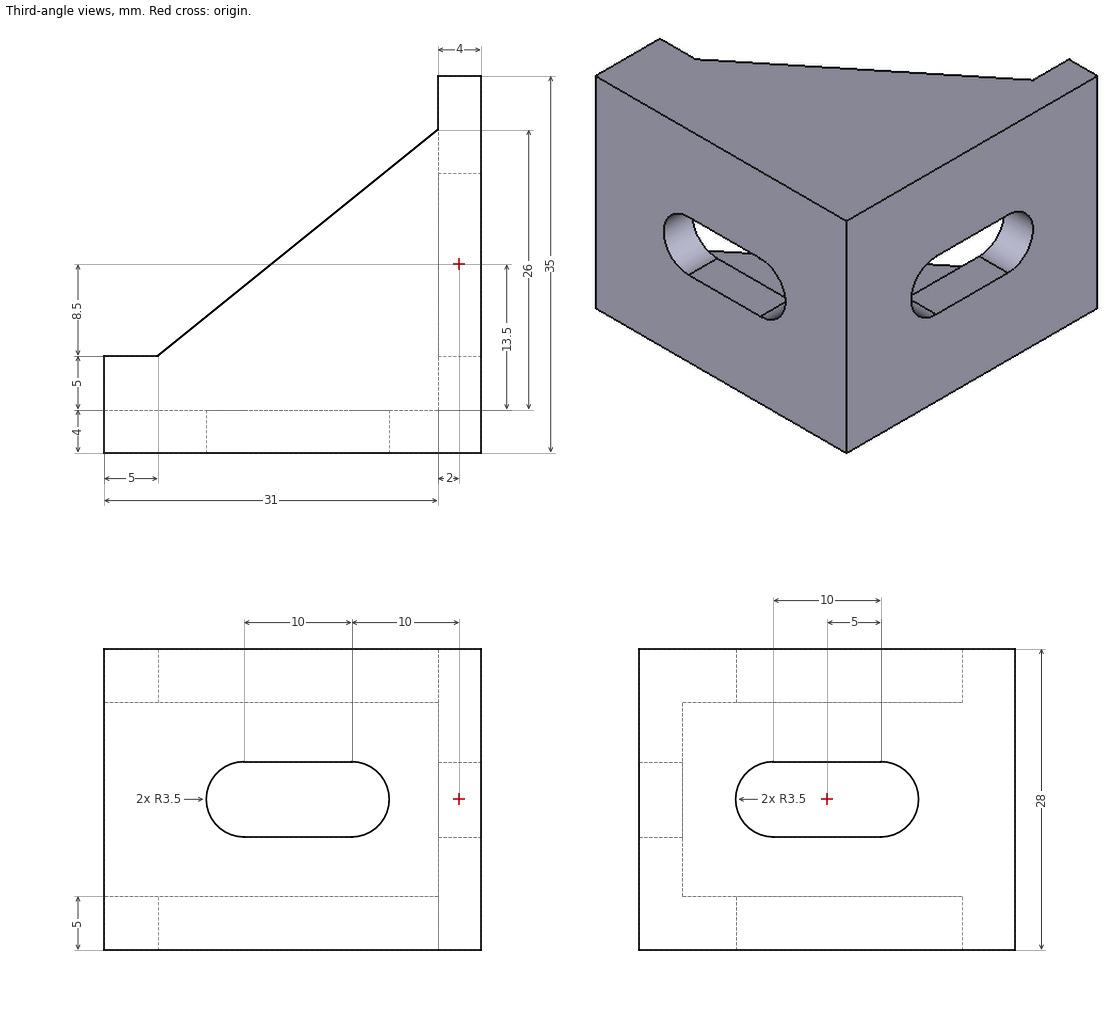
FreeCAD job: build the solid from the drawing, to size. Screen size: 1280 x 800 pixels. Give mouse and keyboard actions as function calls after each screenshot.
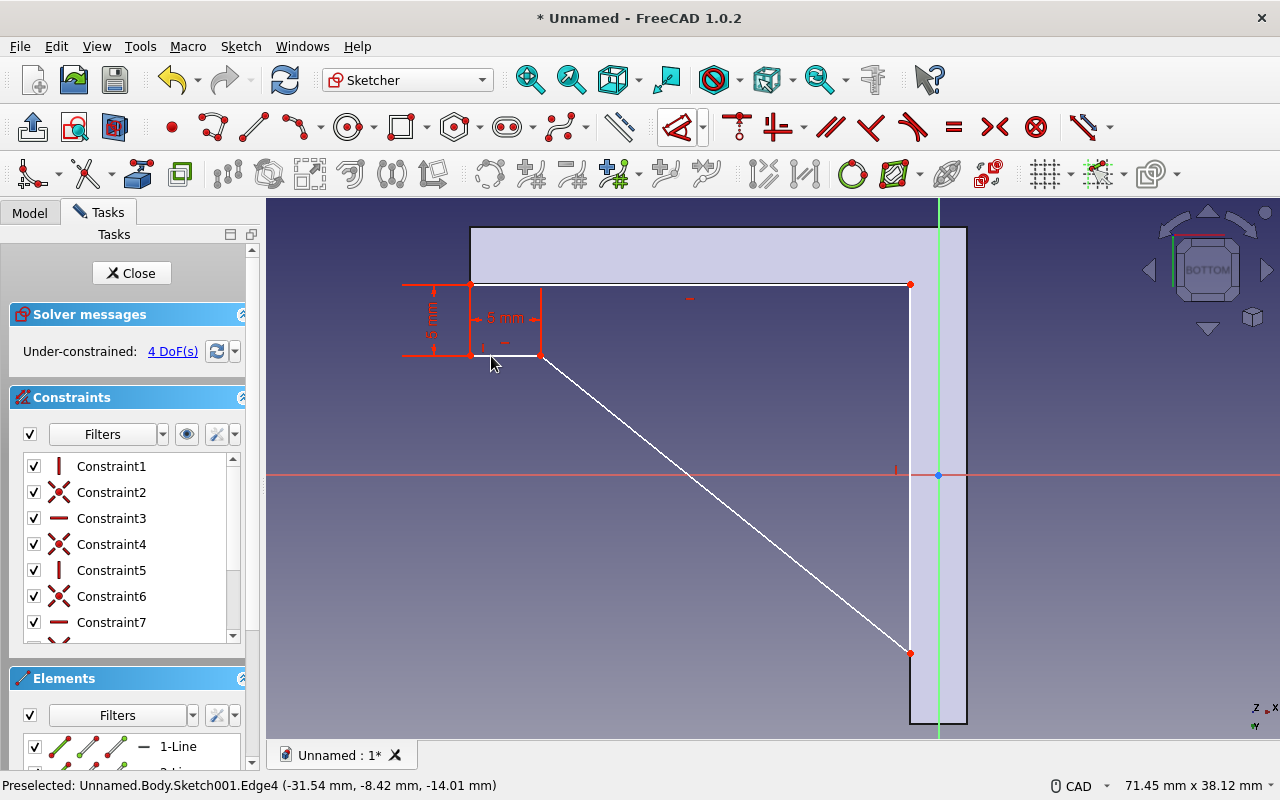
click(910, 543)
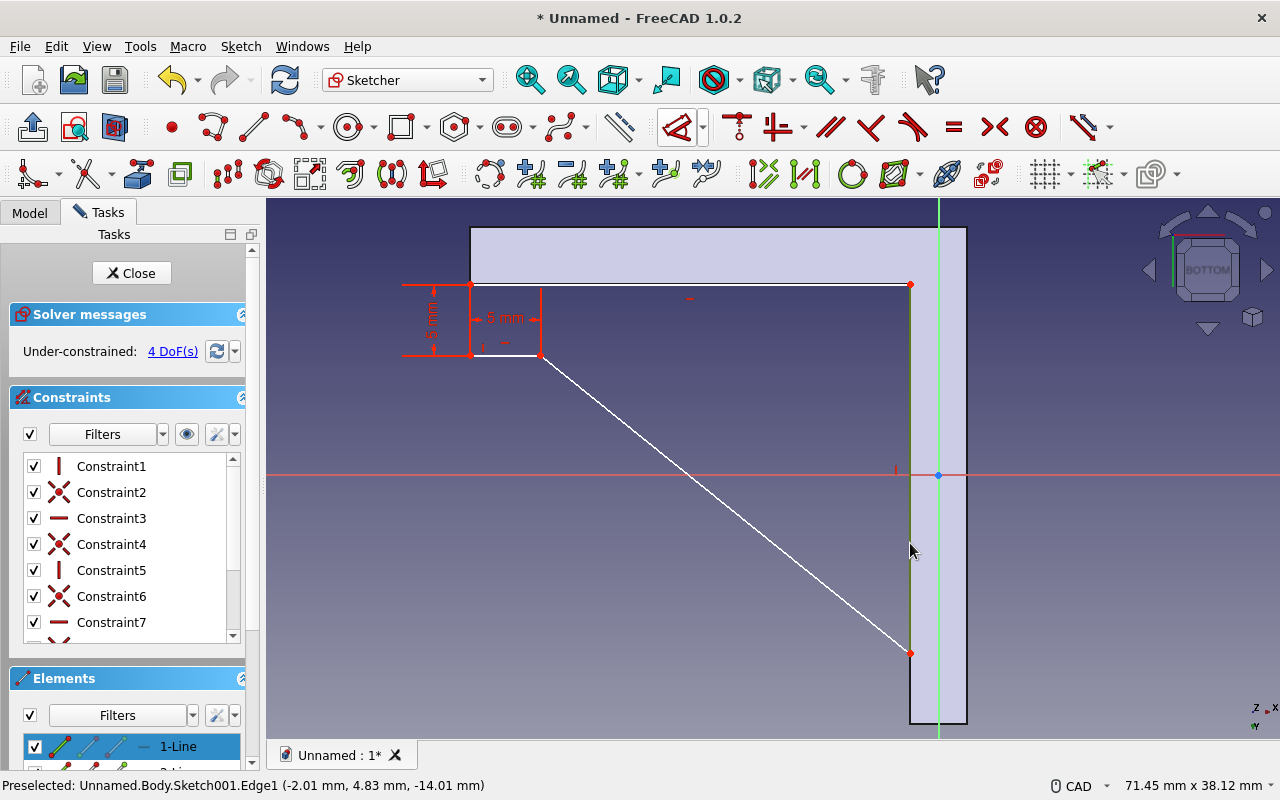
click(702, 128)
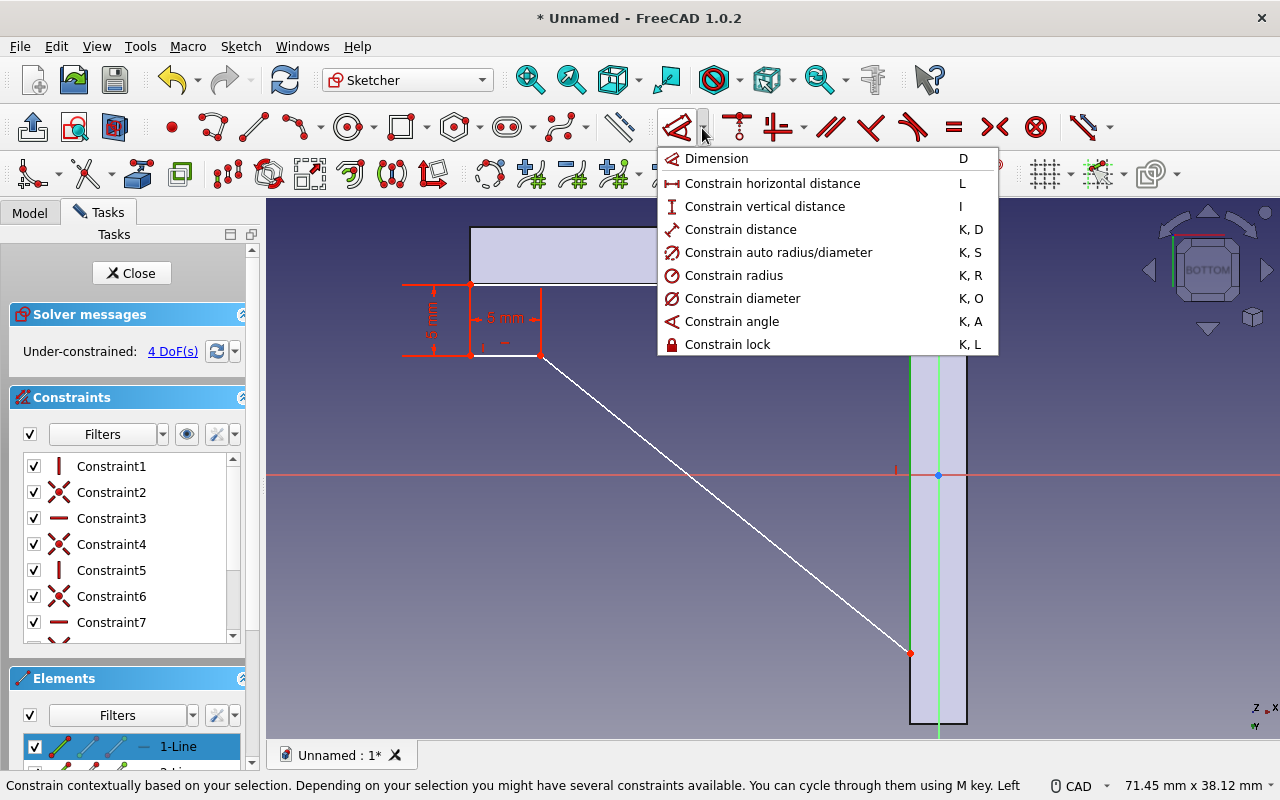
click(828, 206)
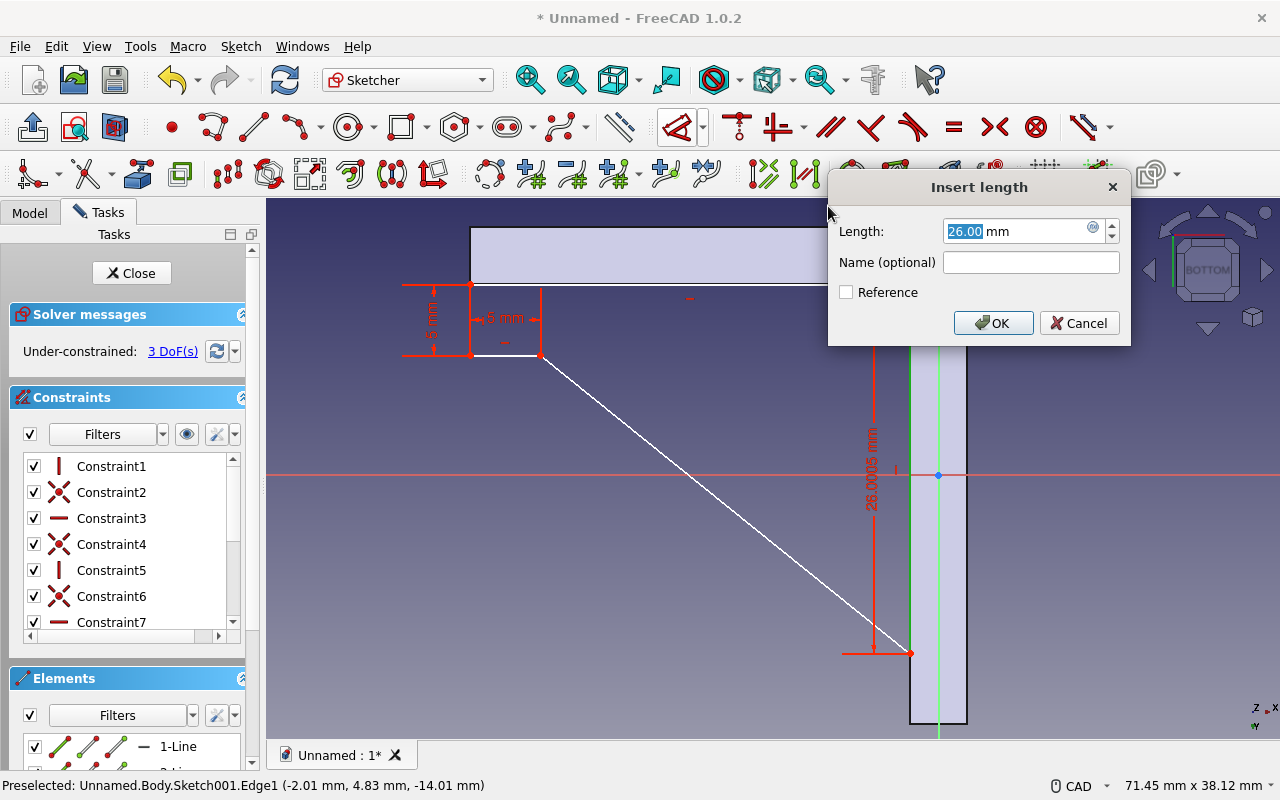
text(26)
key(Return)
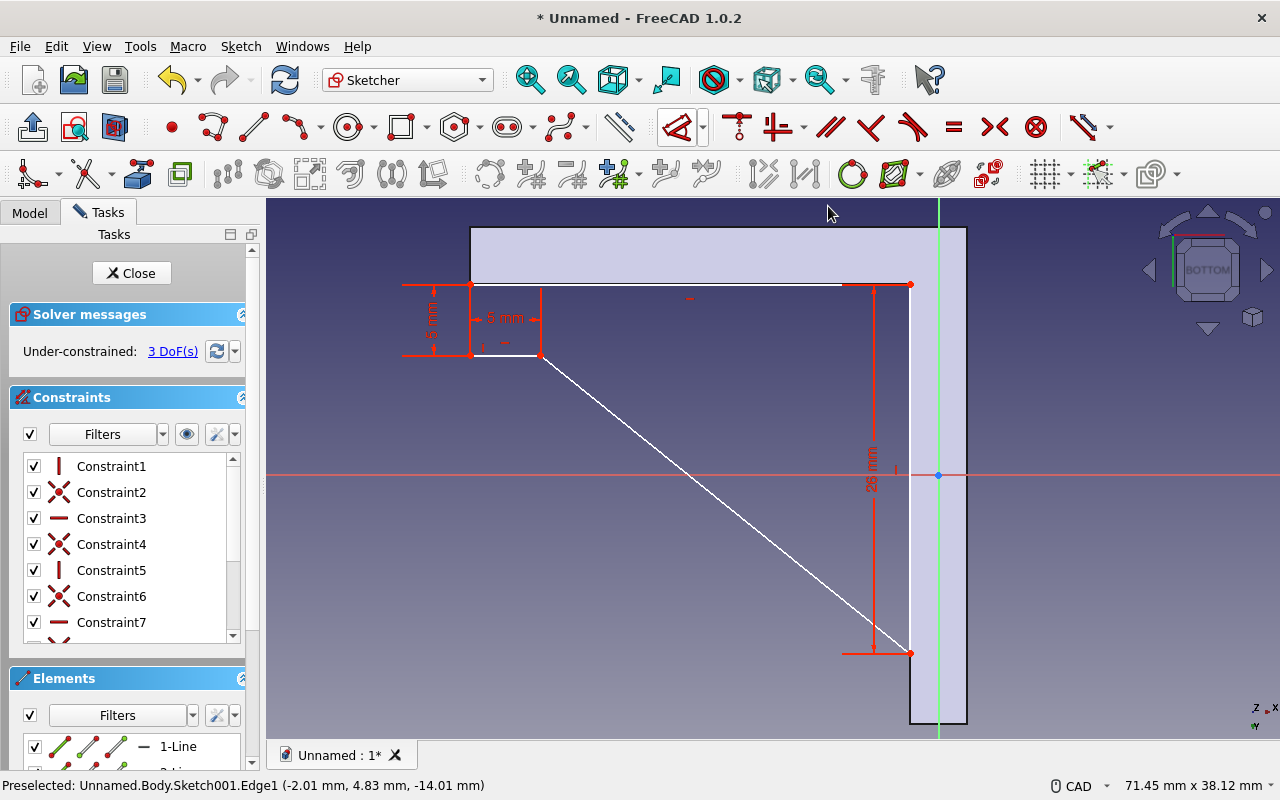
click(778, 285)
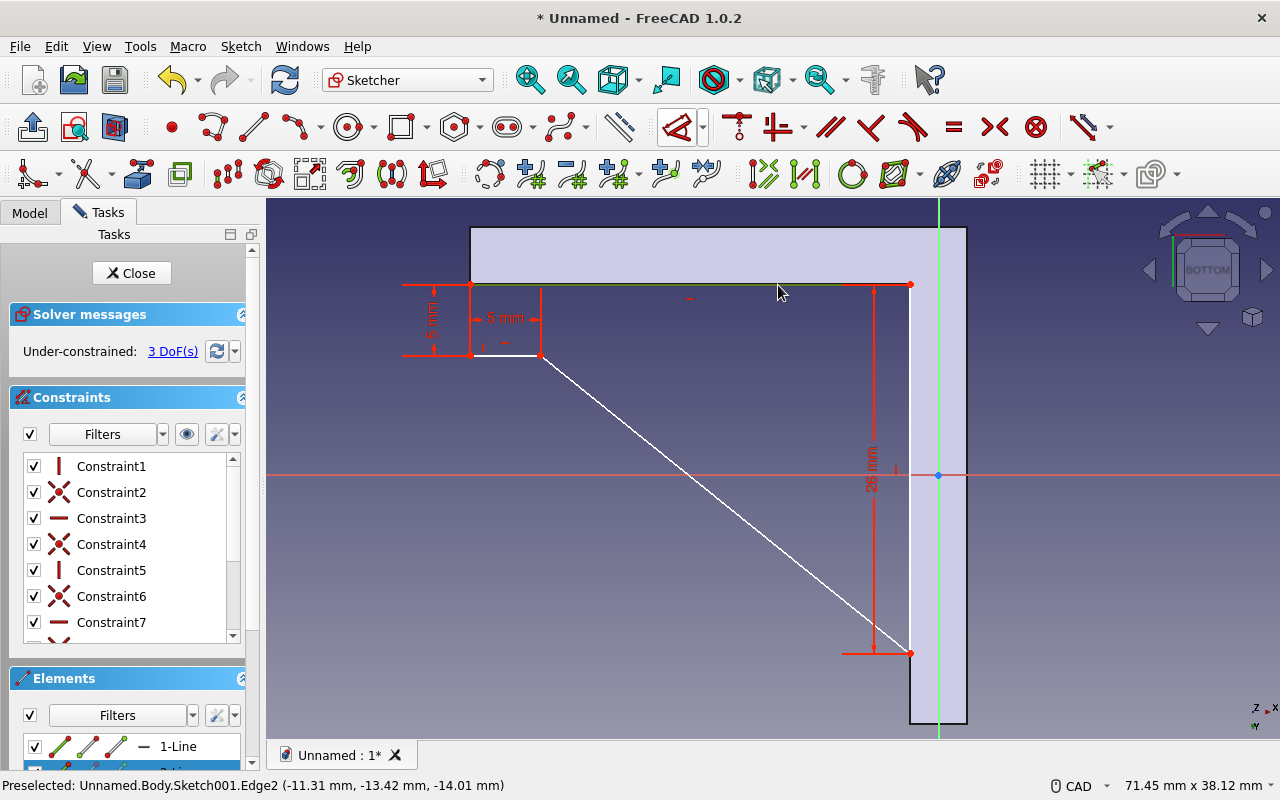
click(702, 128)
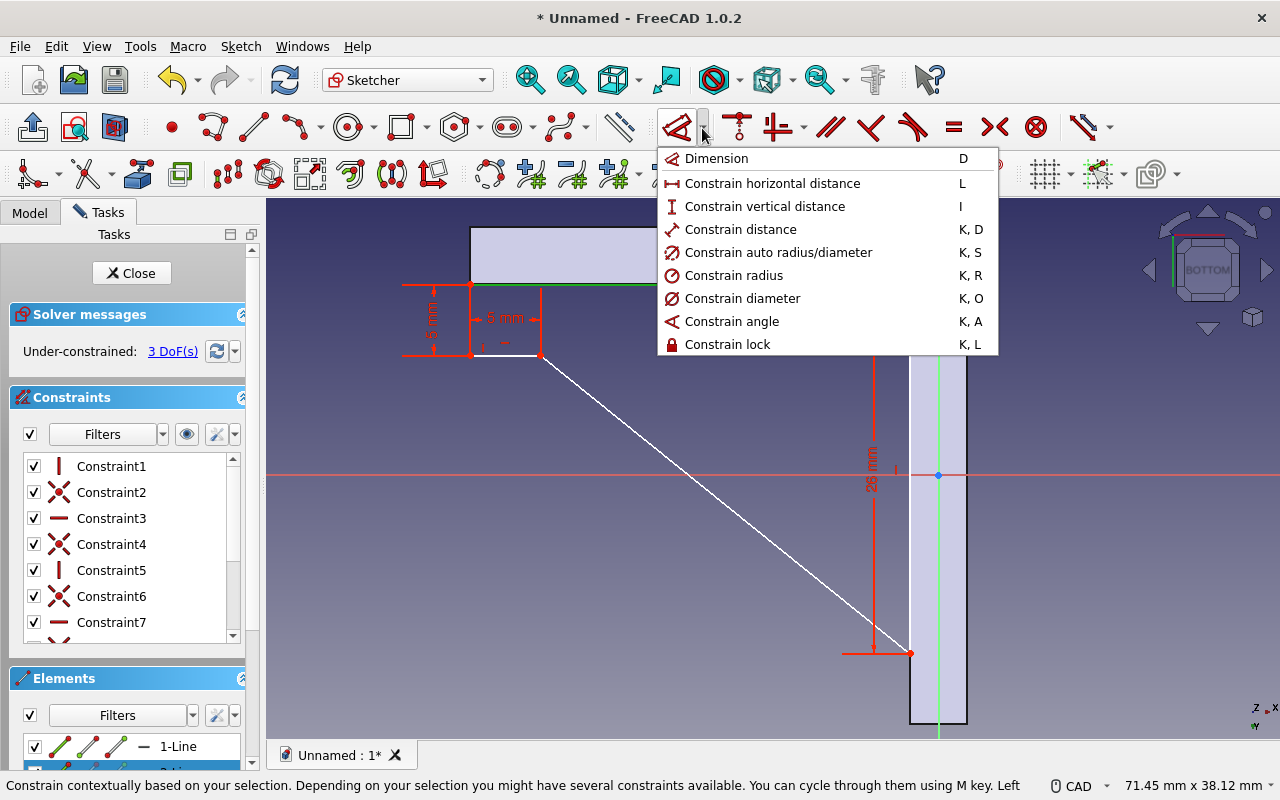
click(828, 184)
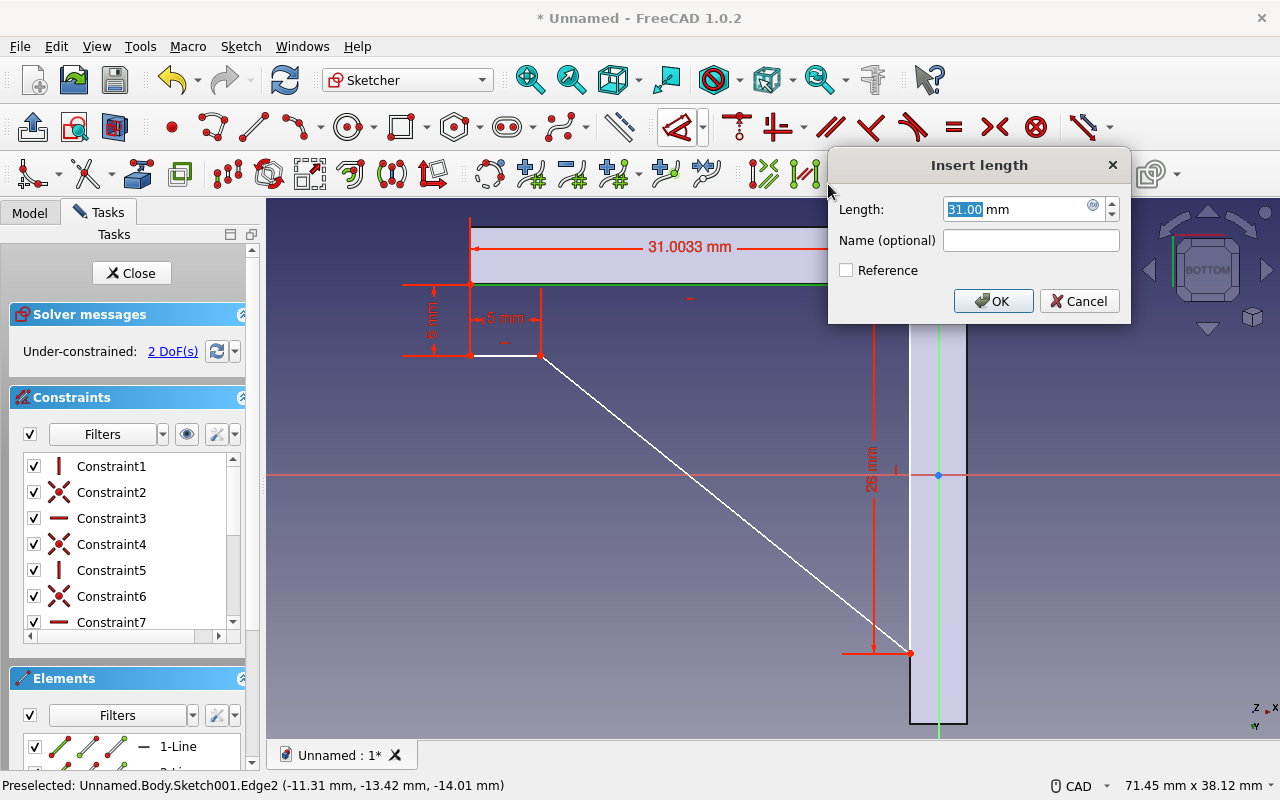
text(31)
key(Return)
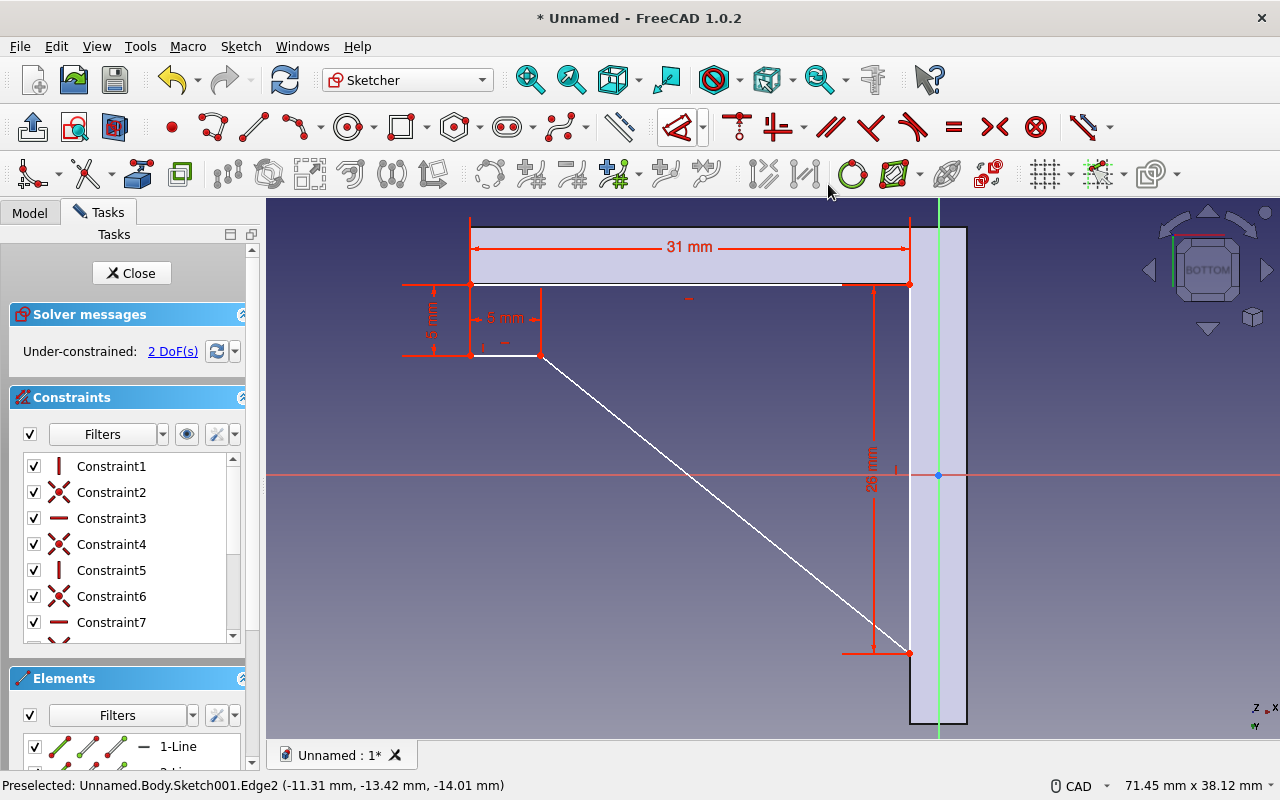
scroll(910, 654, up, 2)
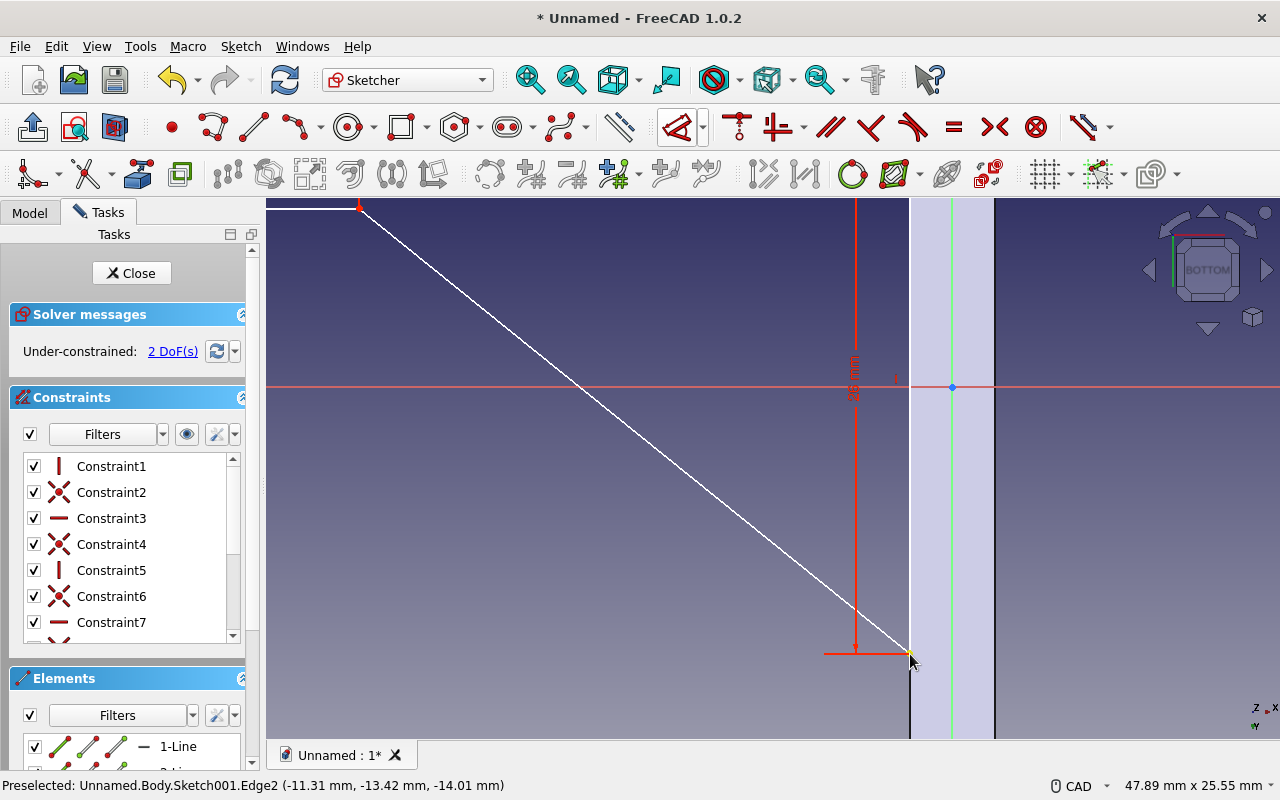
click(910, 654)